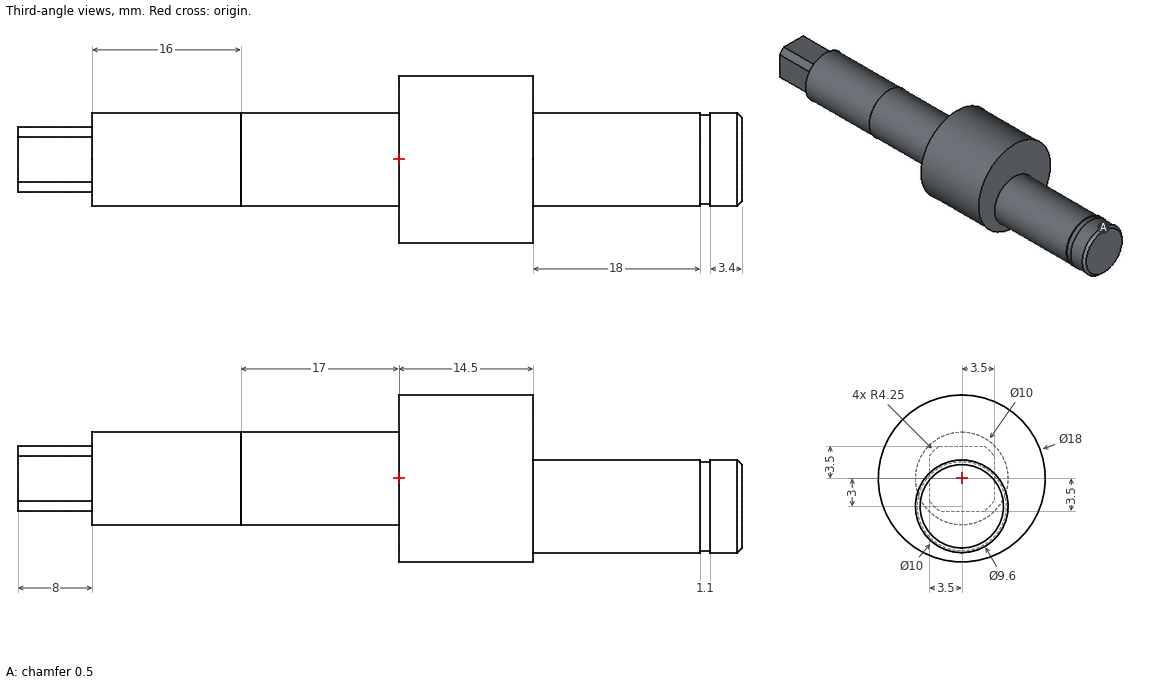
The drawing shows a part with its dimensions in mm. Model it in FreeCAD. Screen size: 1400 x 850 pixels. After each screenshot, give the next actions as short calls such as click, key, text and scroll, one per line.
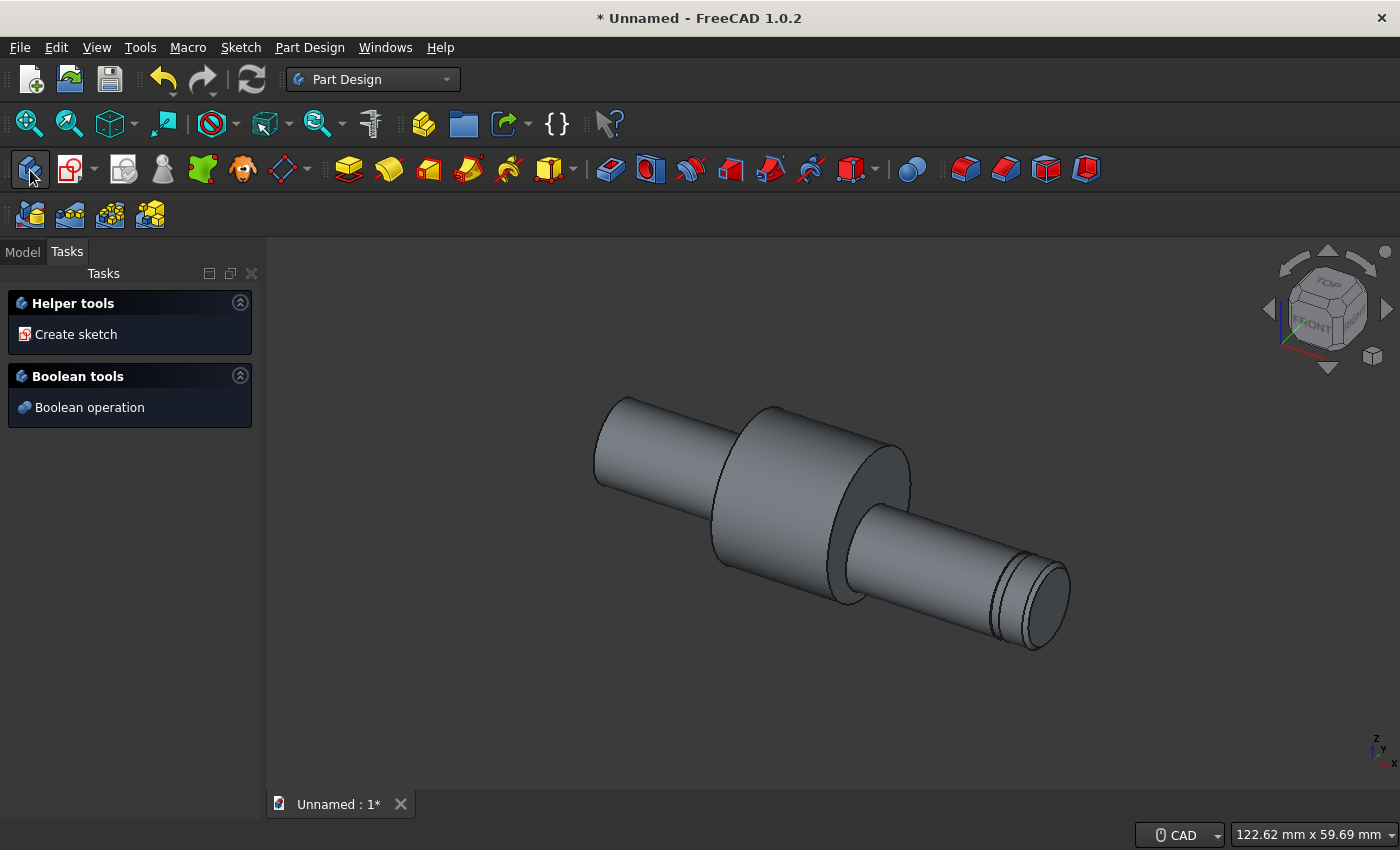
click(23, 251)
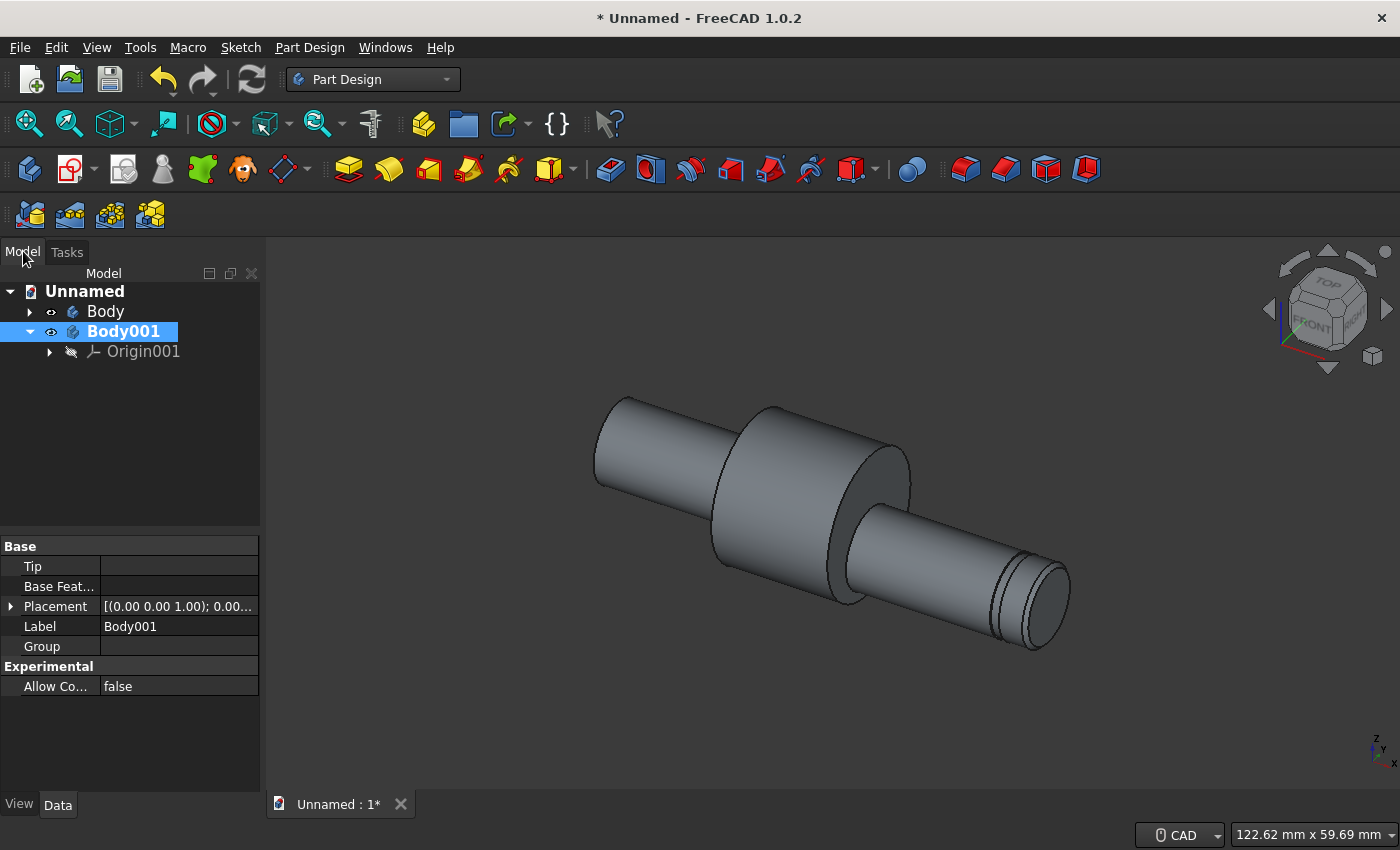
click(50, 352)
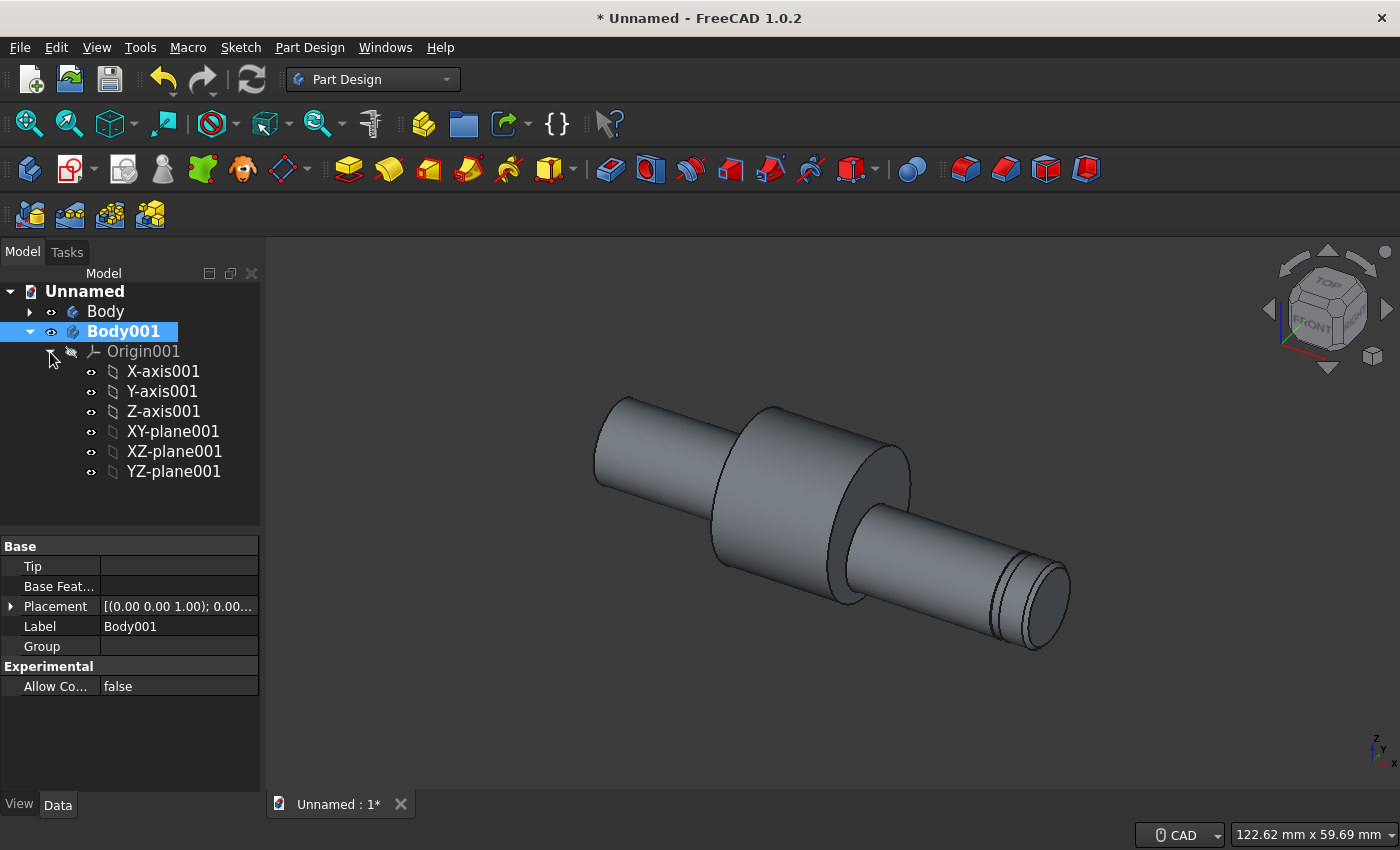
click(136, 472)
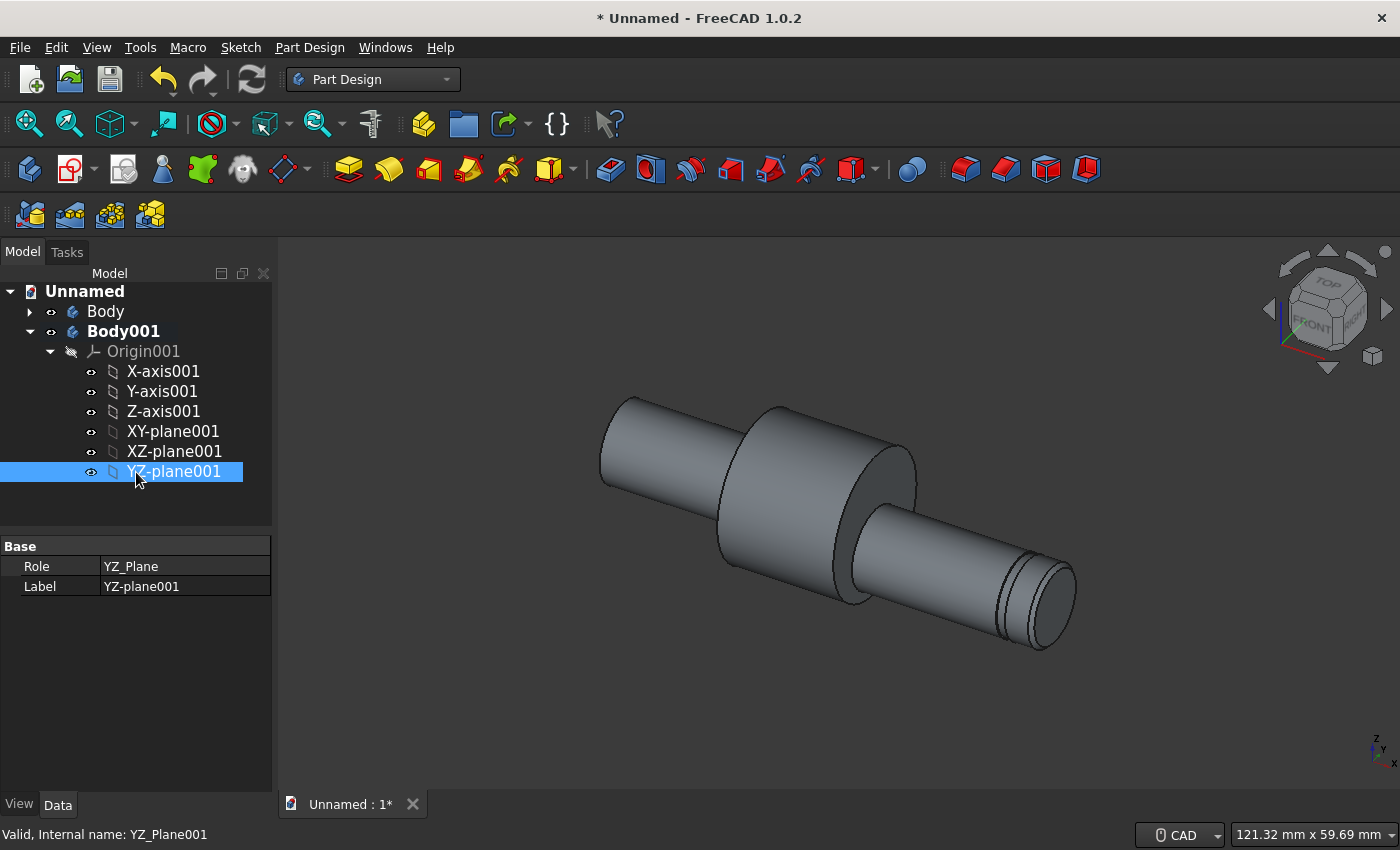
click(284, 170)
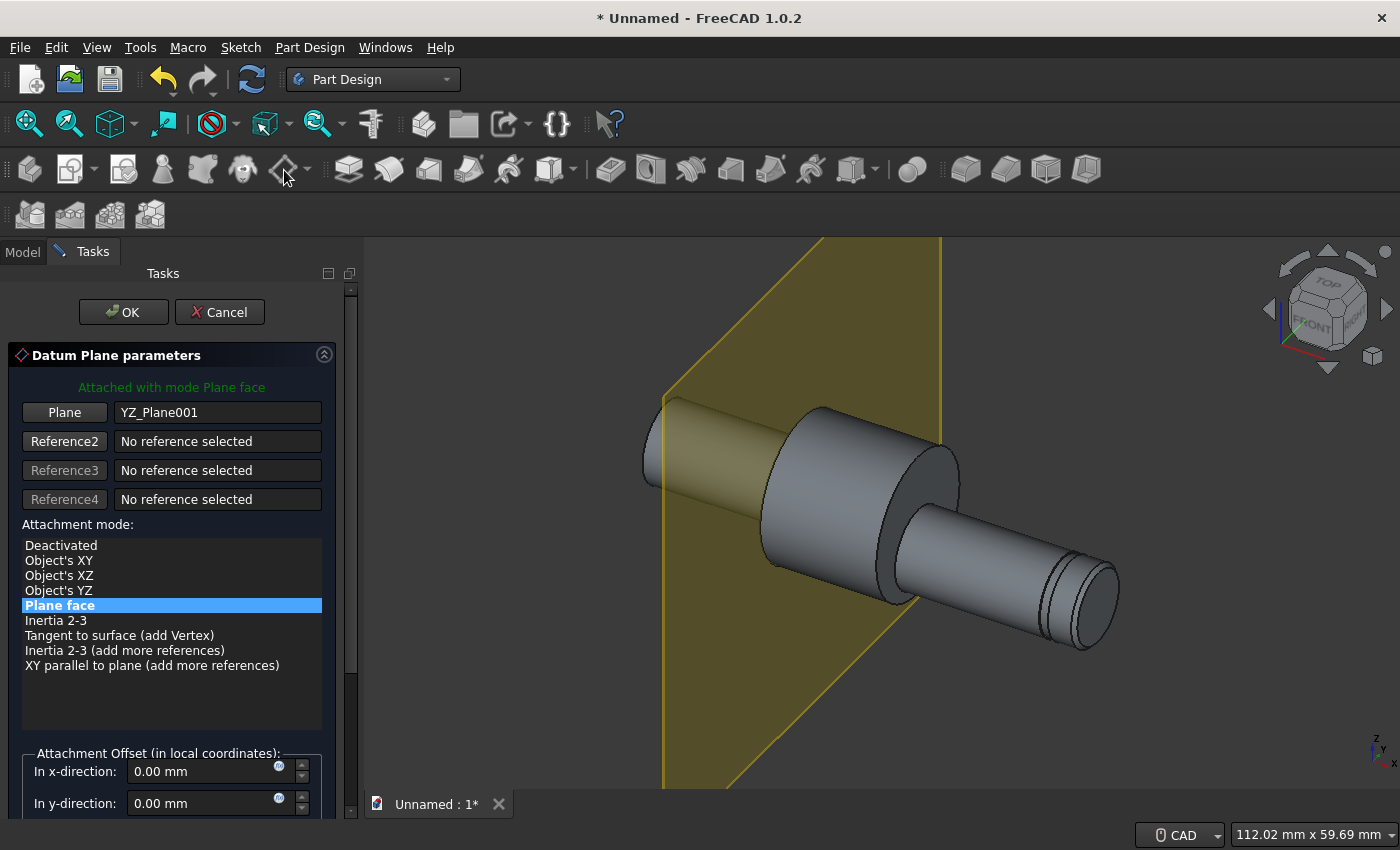
scroll(351, 550, down, 2)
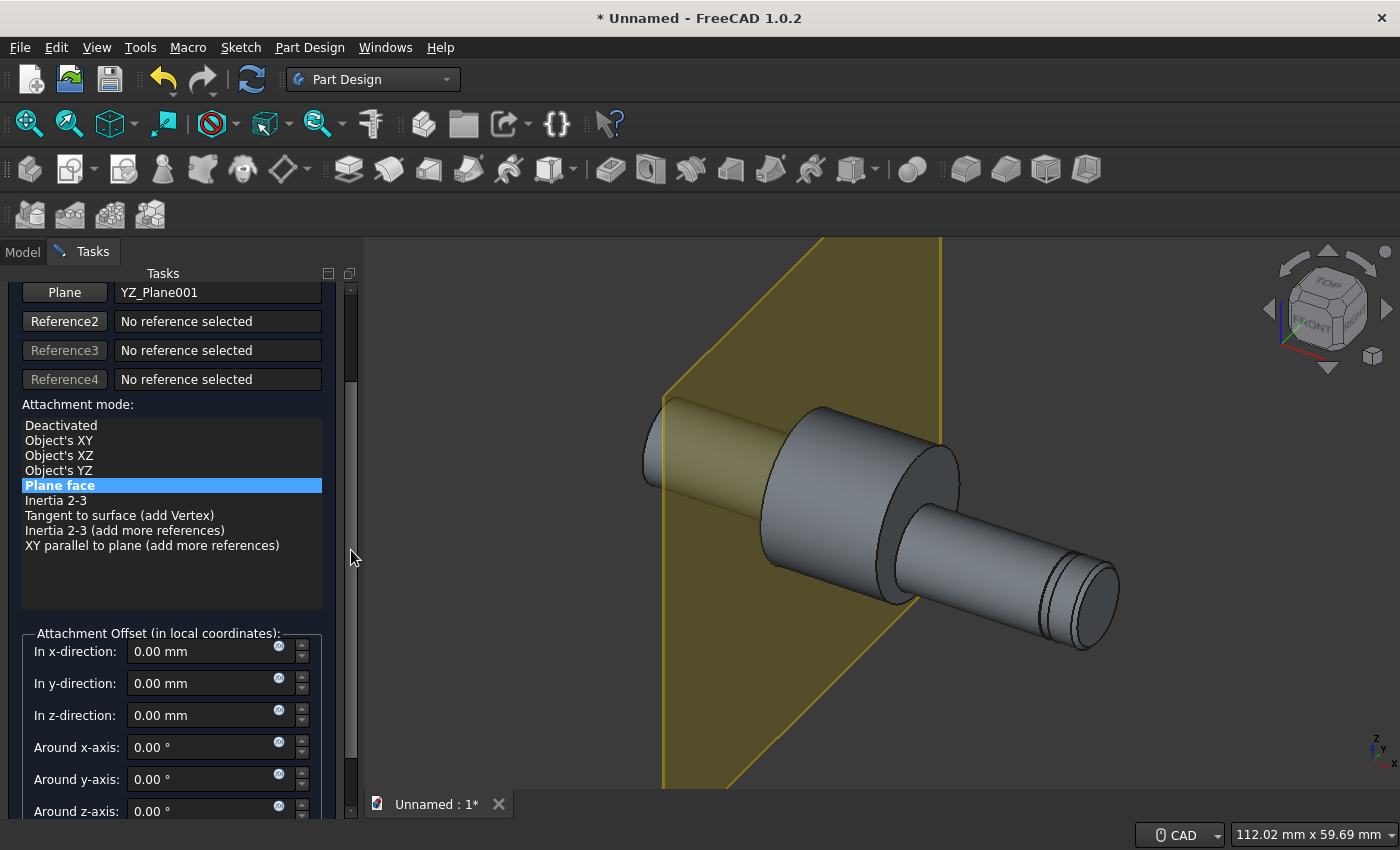
triple_click(210, 715)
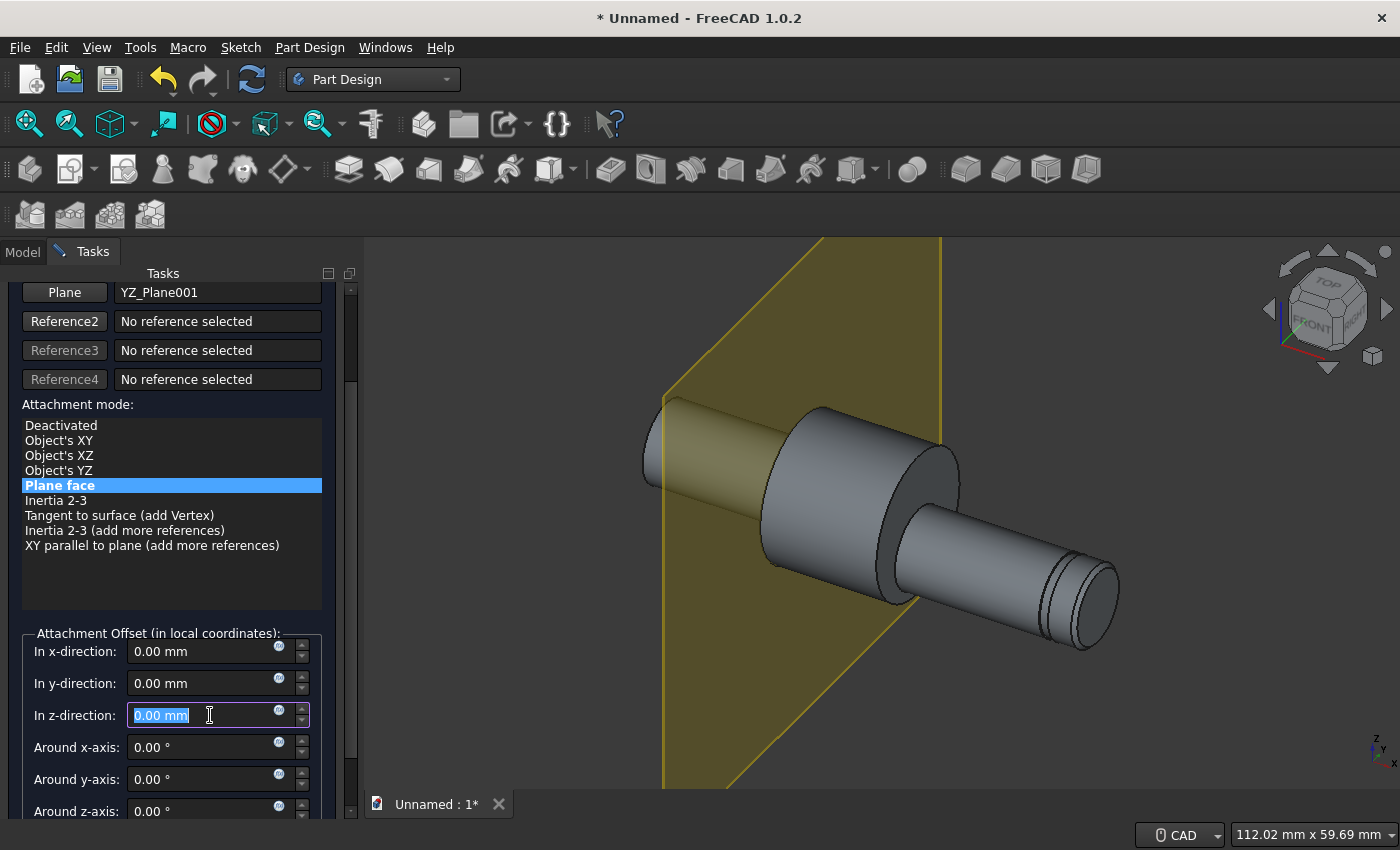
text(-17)
key(Tab)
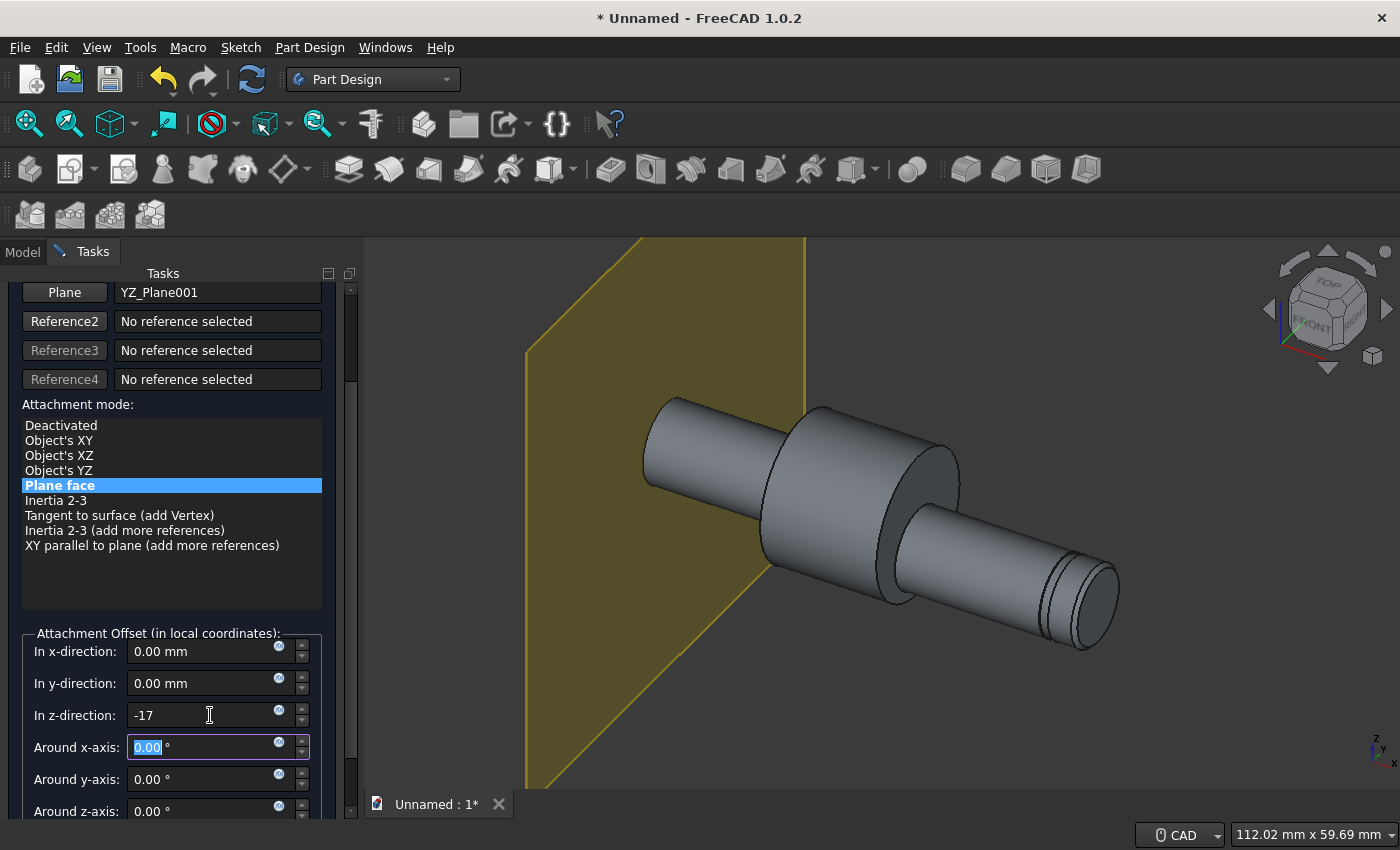
scroll(351, 550, up, 3)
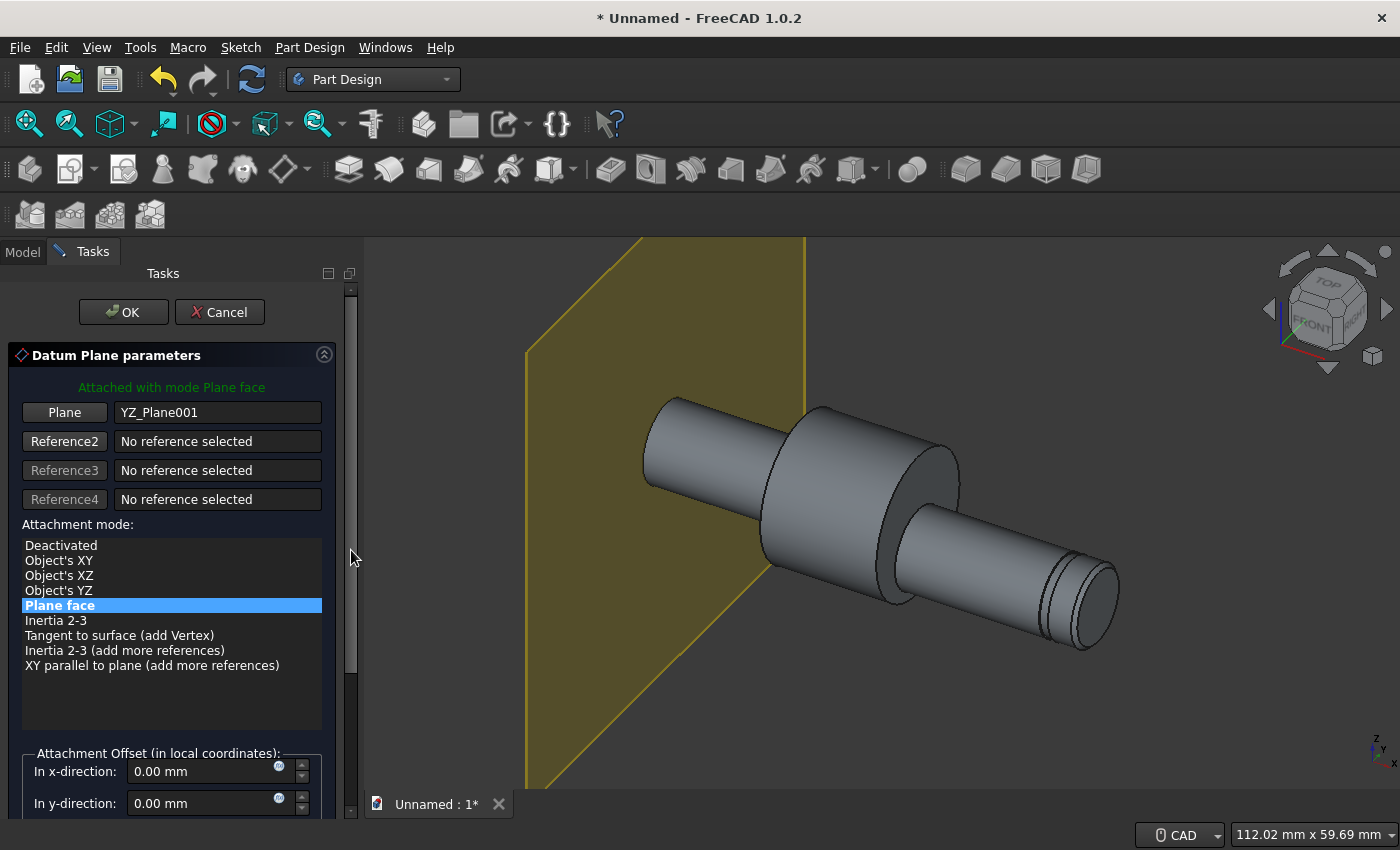
click(124, 312)